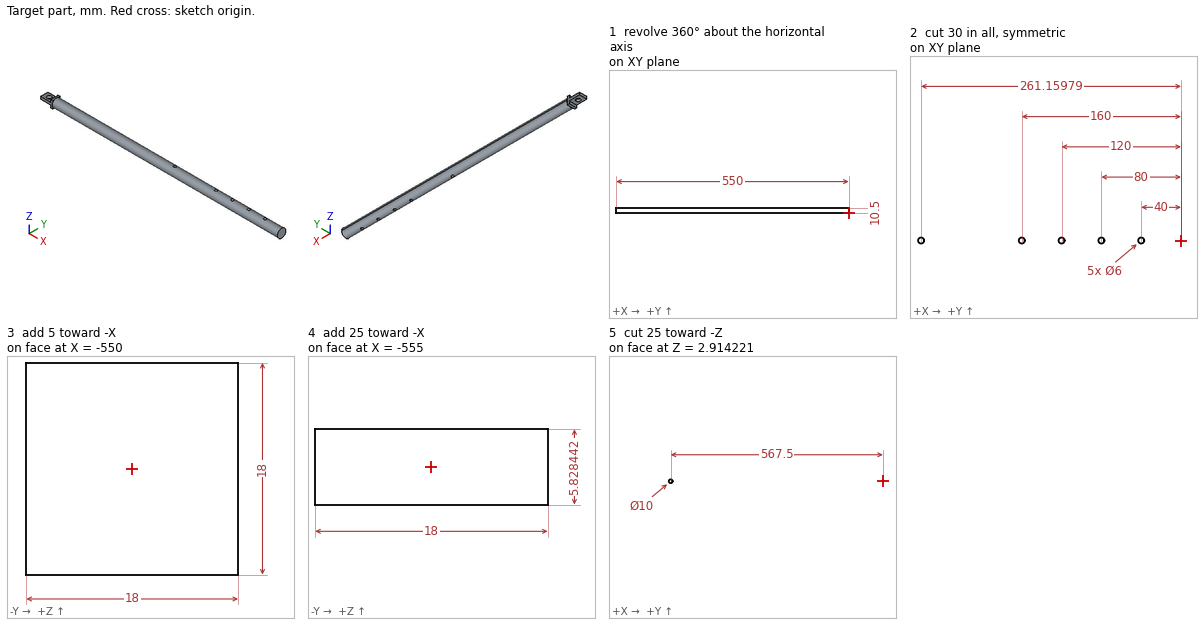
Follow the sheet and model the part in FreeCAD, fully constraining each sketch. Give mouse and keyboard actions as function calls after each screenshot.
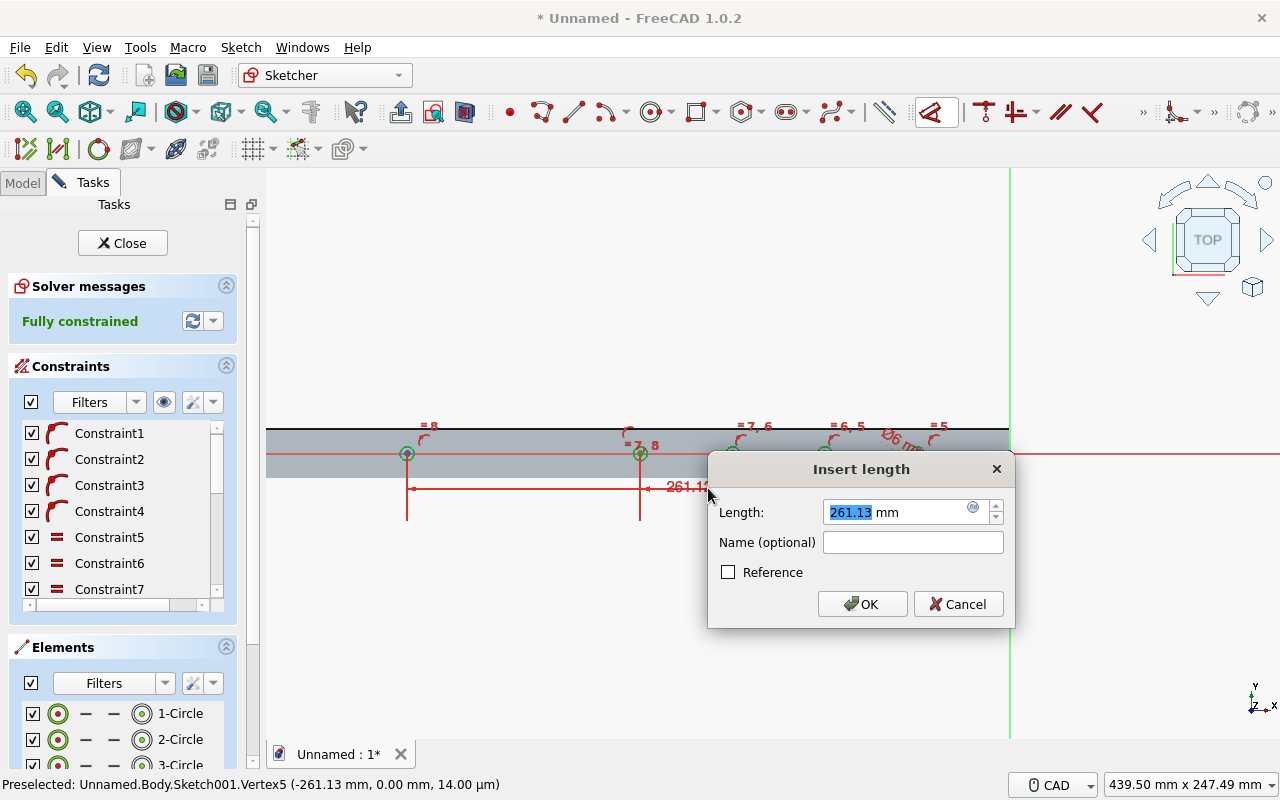
text(261.15979)
key(Return)
key(Escape)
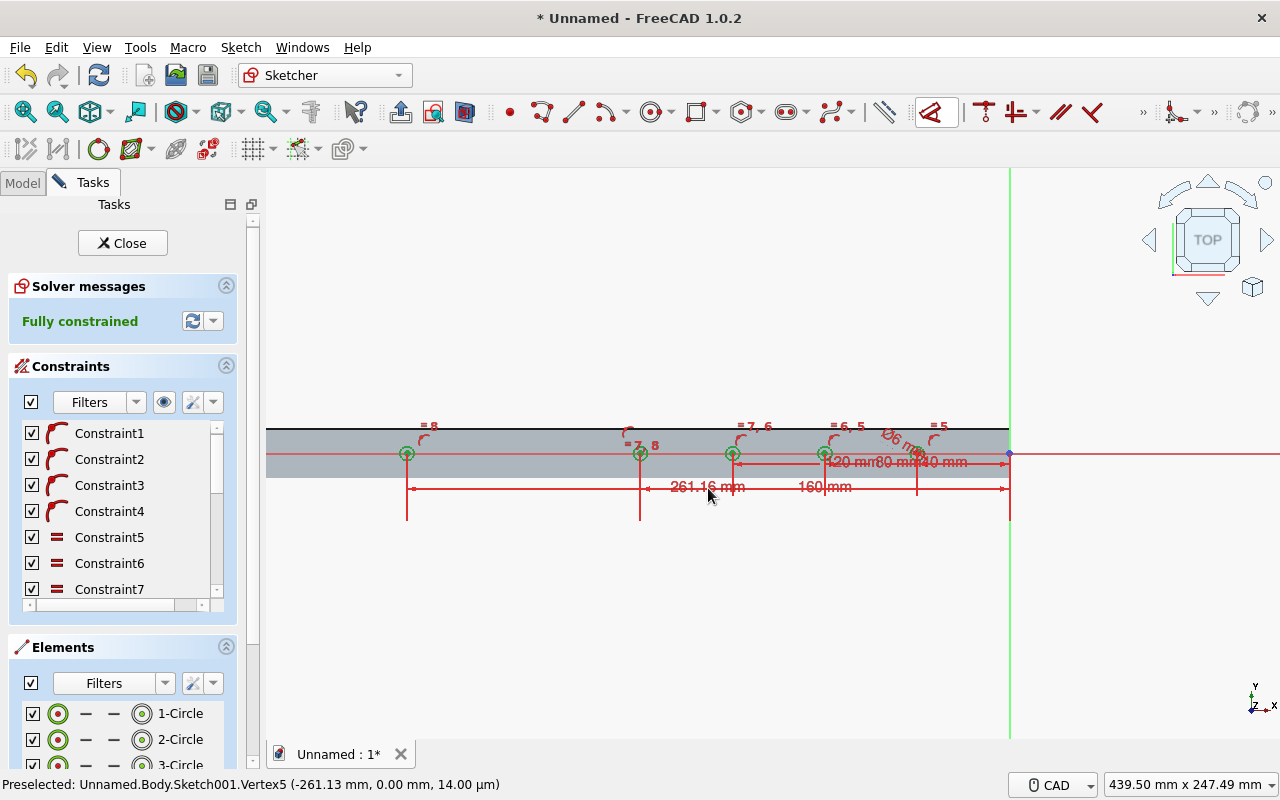
click(123, 243)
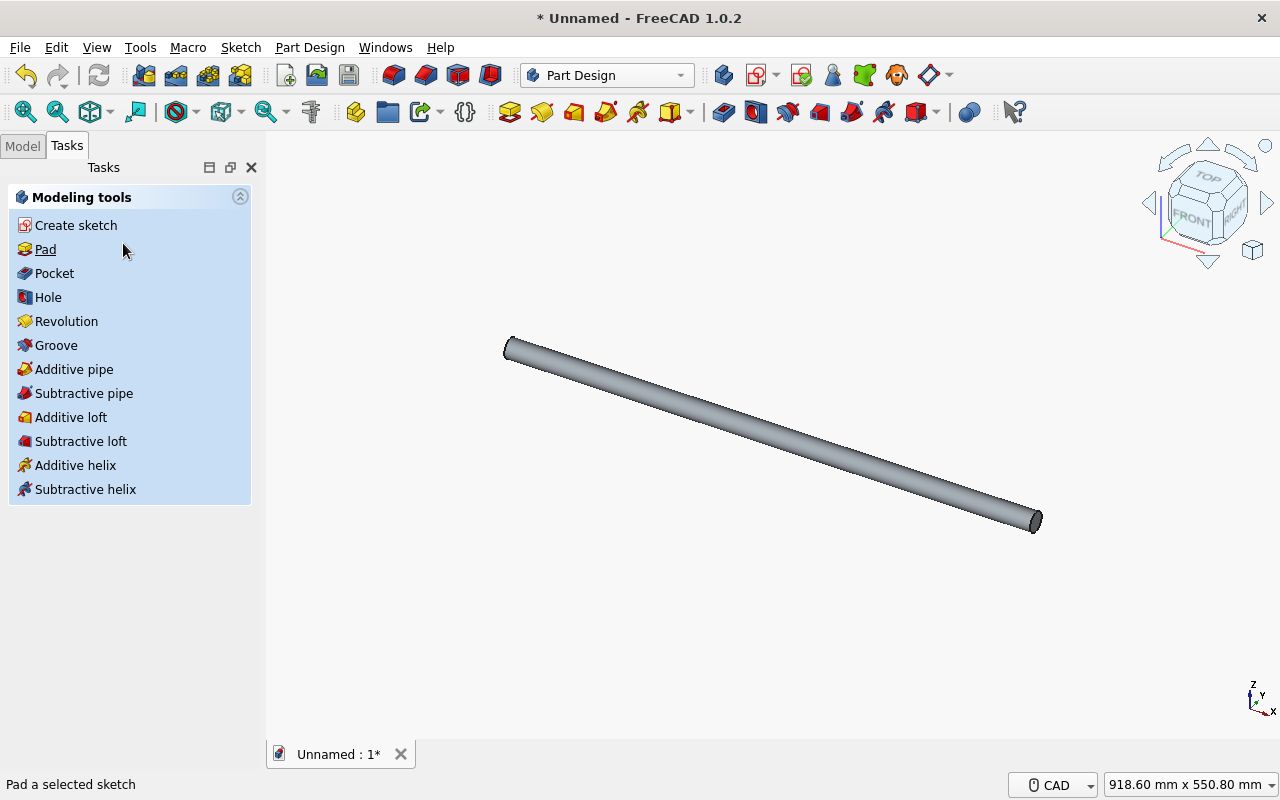
click(724, 112)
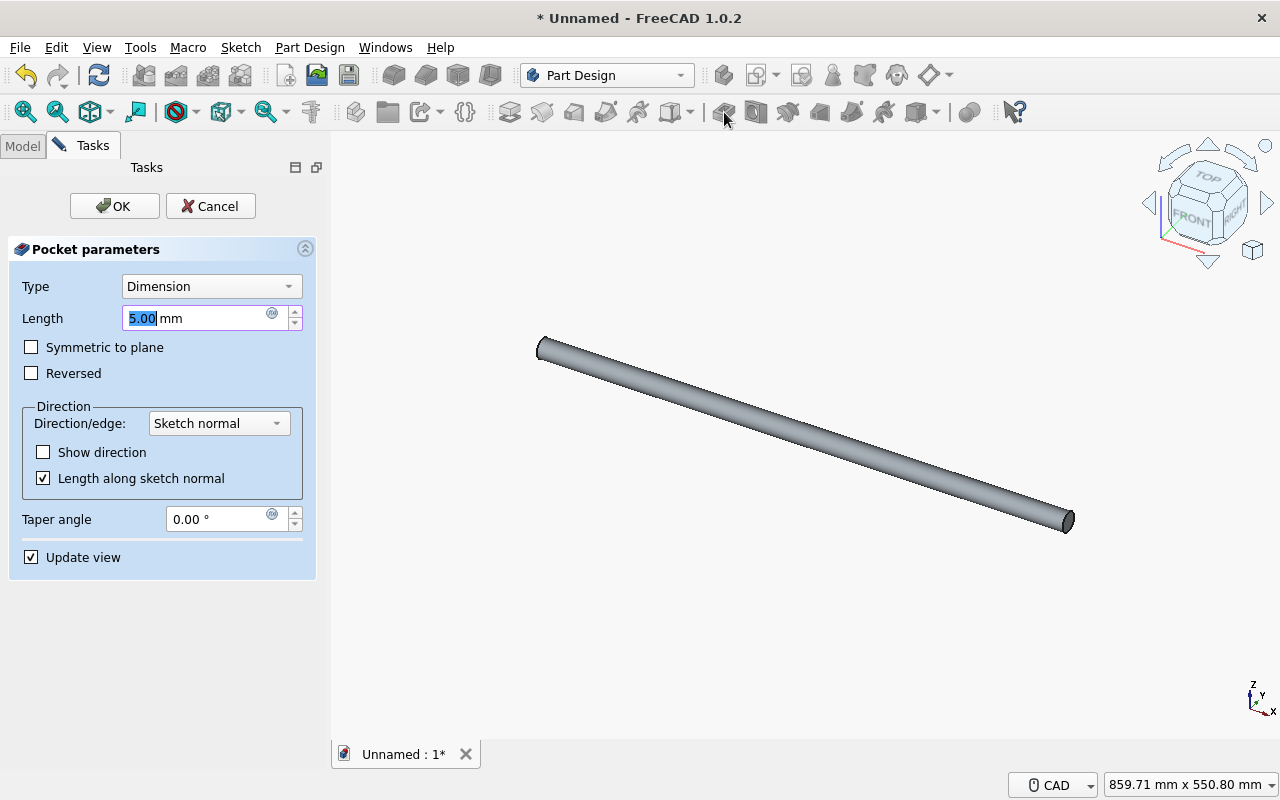
text(30)
key(Tab)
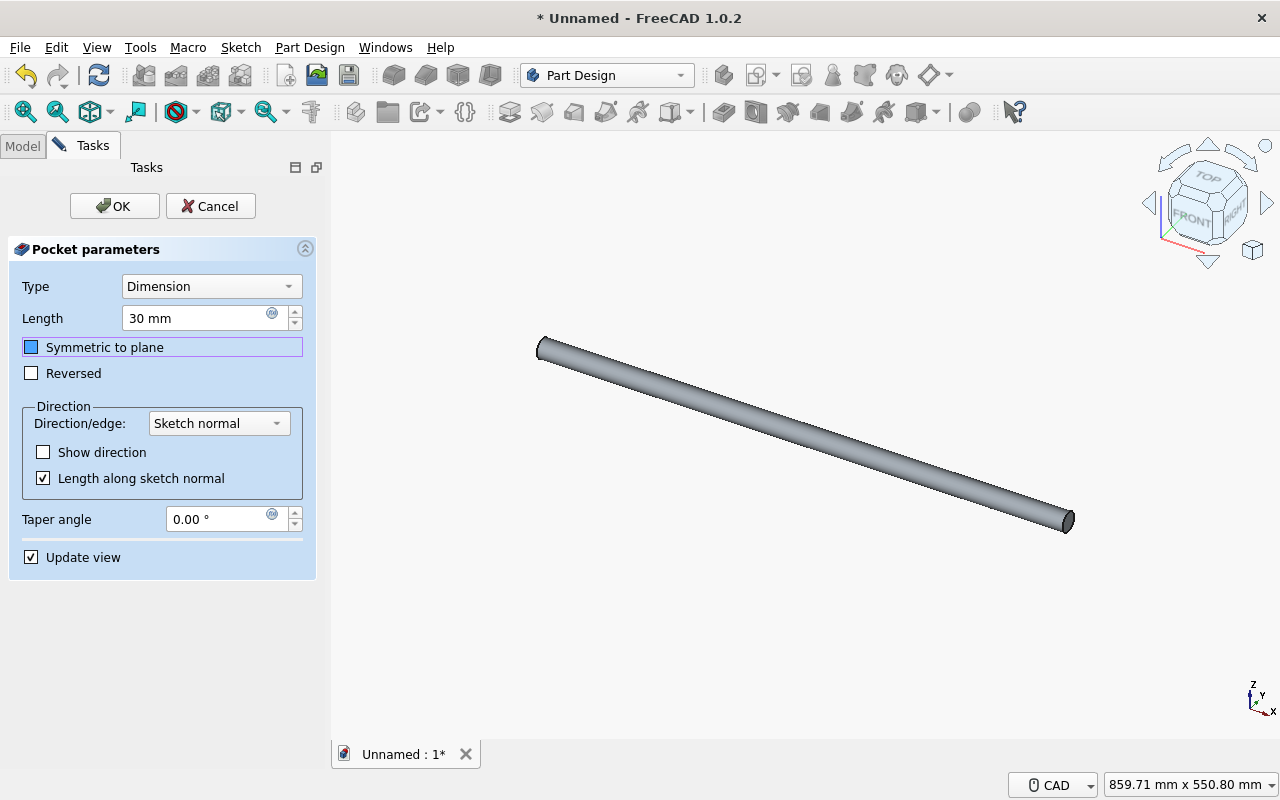
click(30, 347)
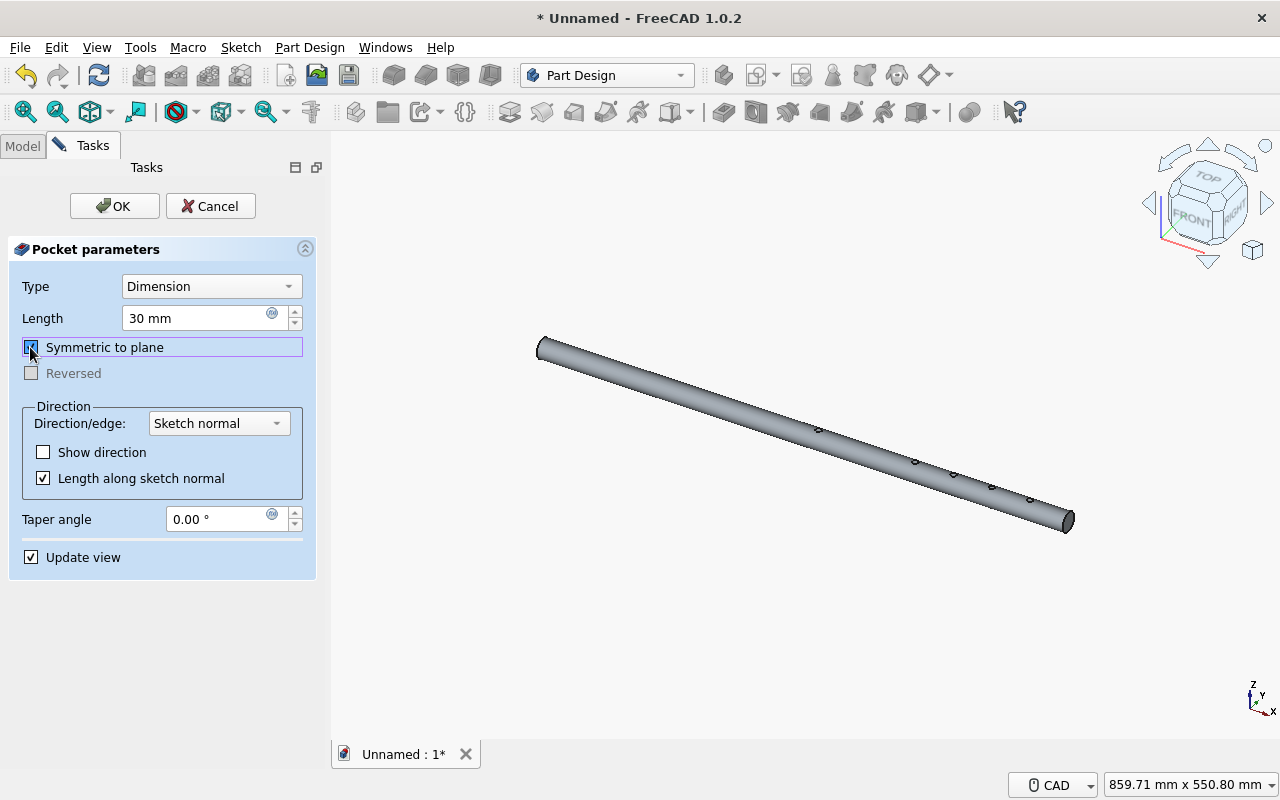
click(115, 206)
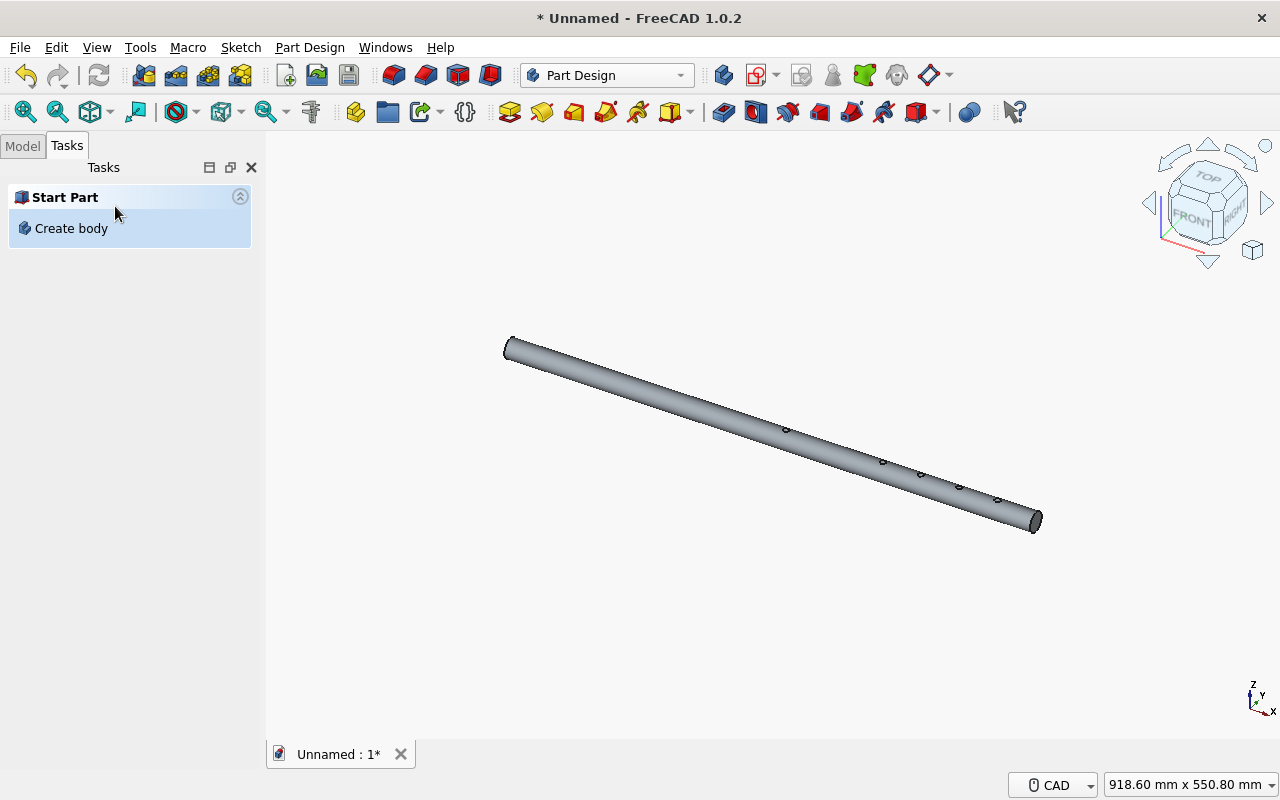
key(6)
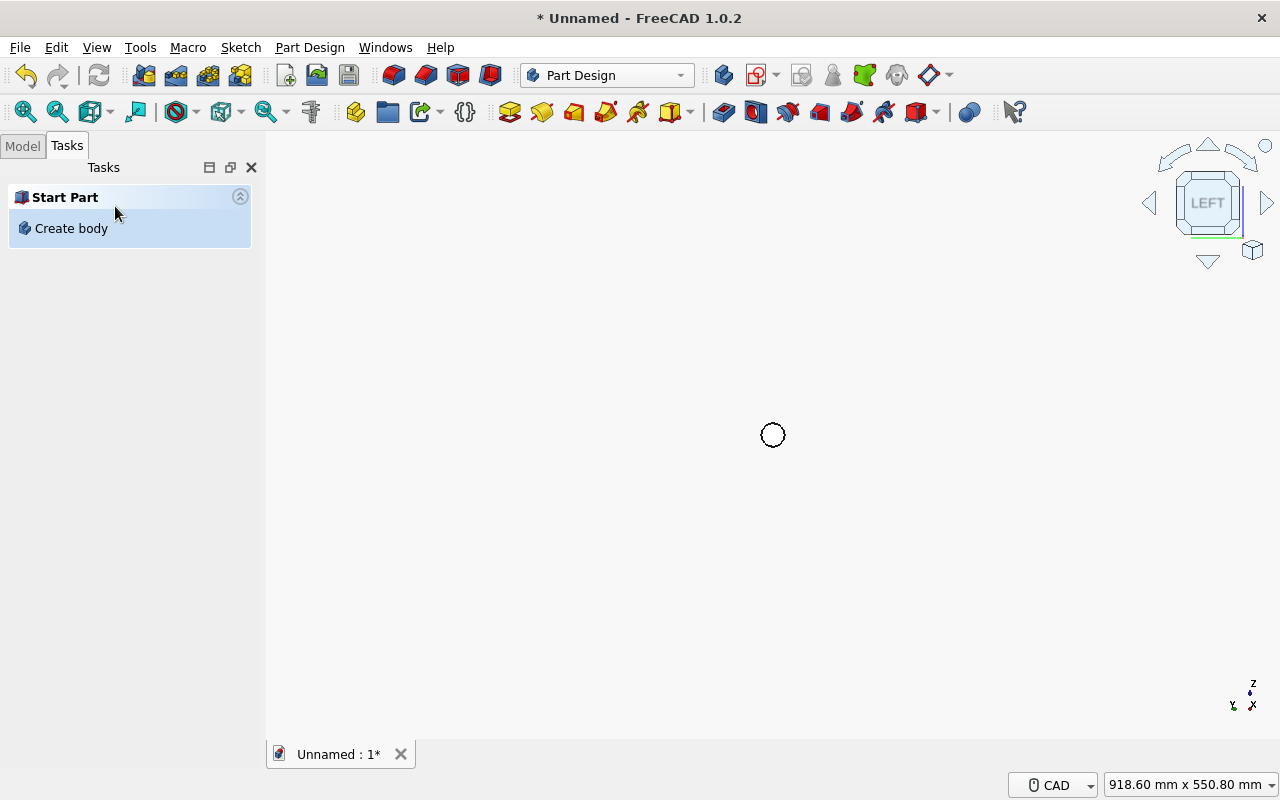
key(v)
key(f)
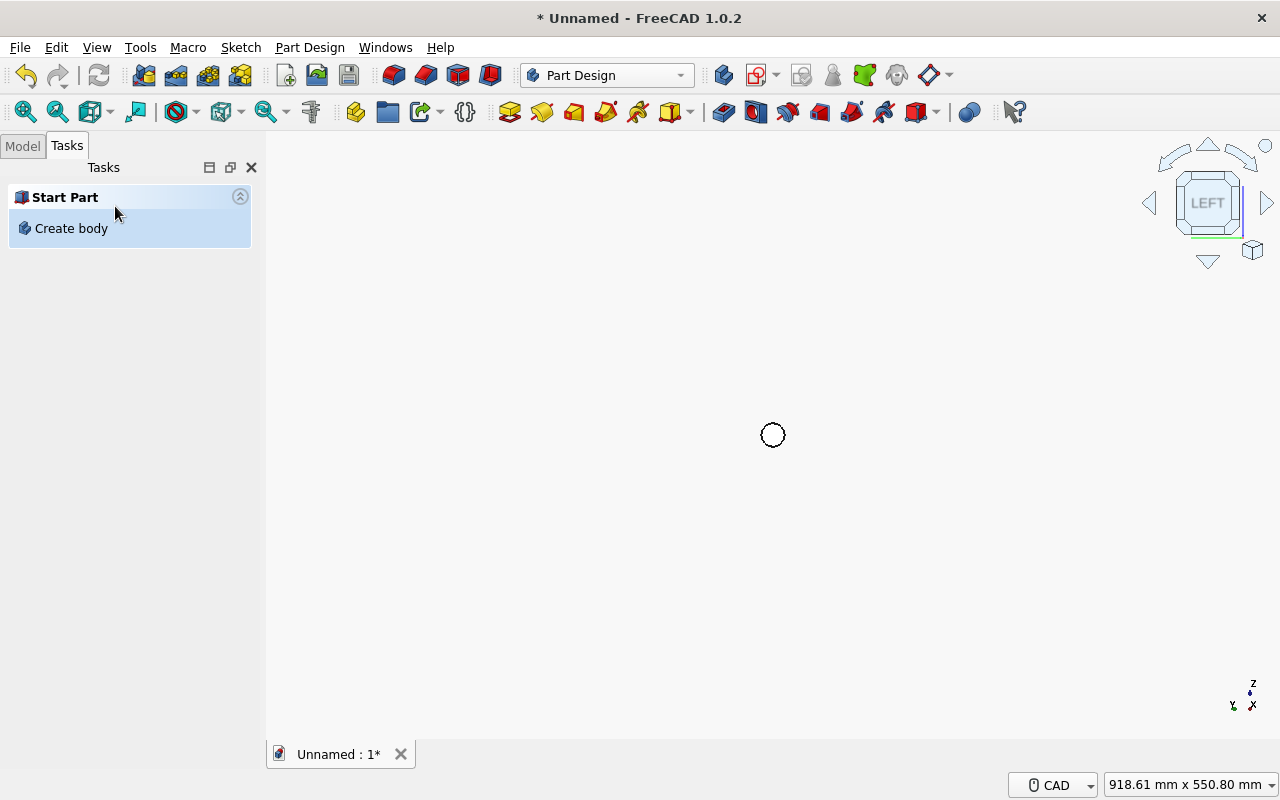
click(773, 434)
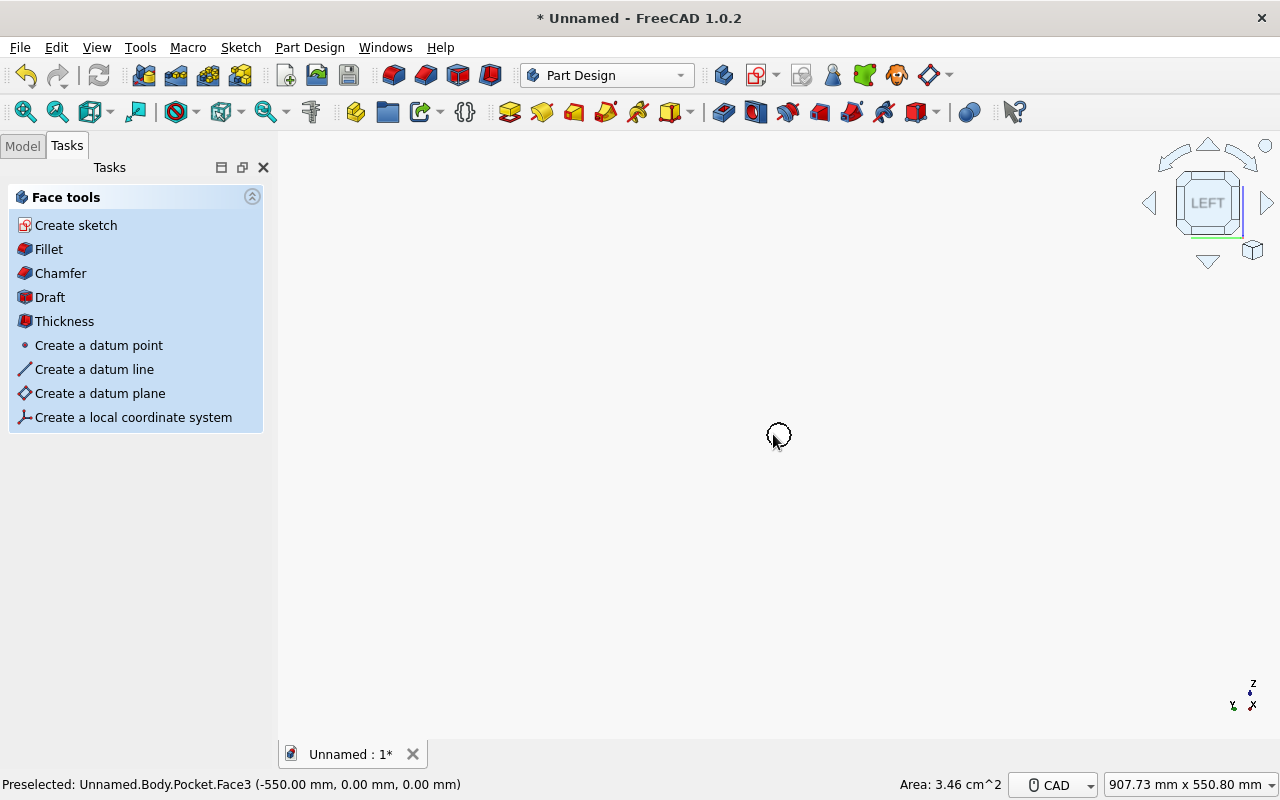
click(756, 76)